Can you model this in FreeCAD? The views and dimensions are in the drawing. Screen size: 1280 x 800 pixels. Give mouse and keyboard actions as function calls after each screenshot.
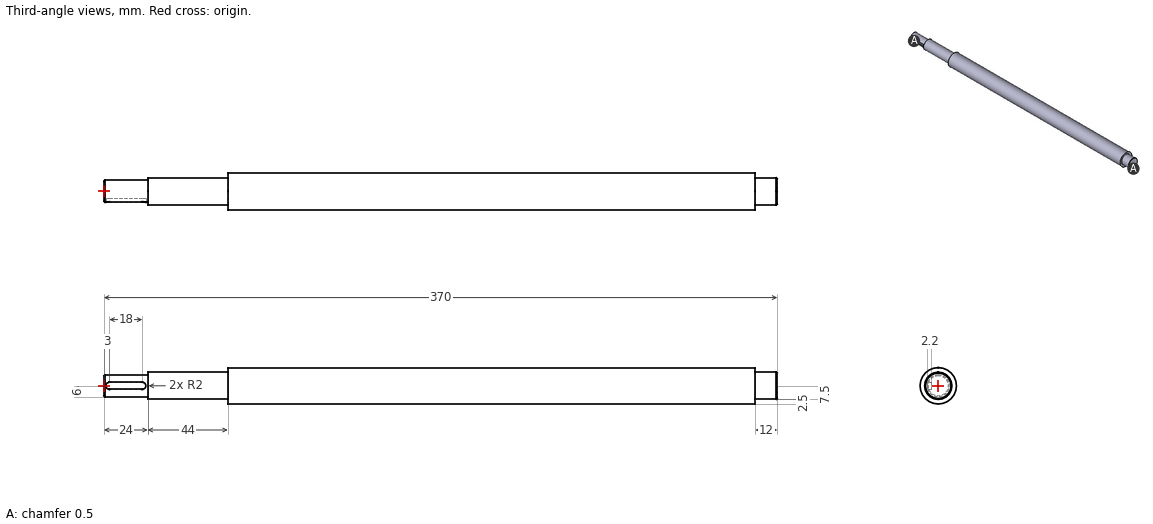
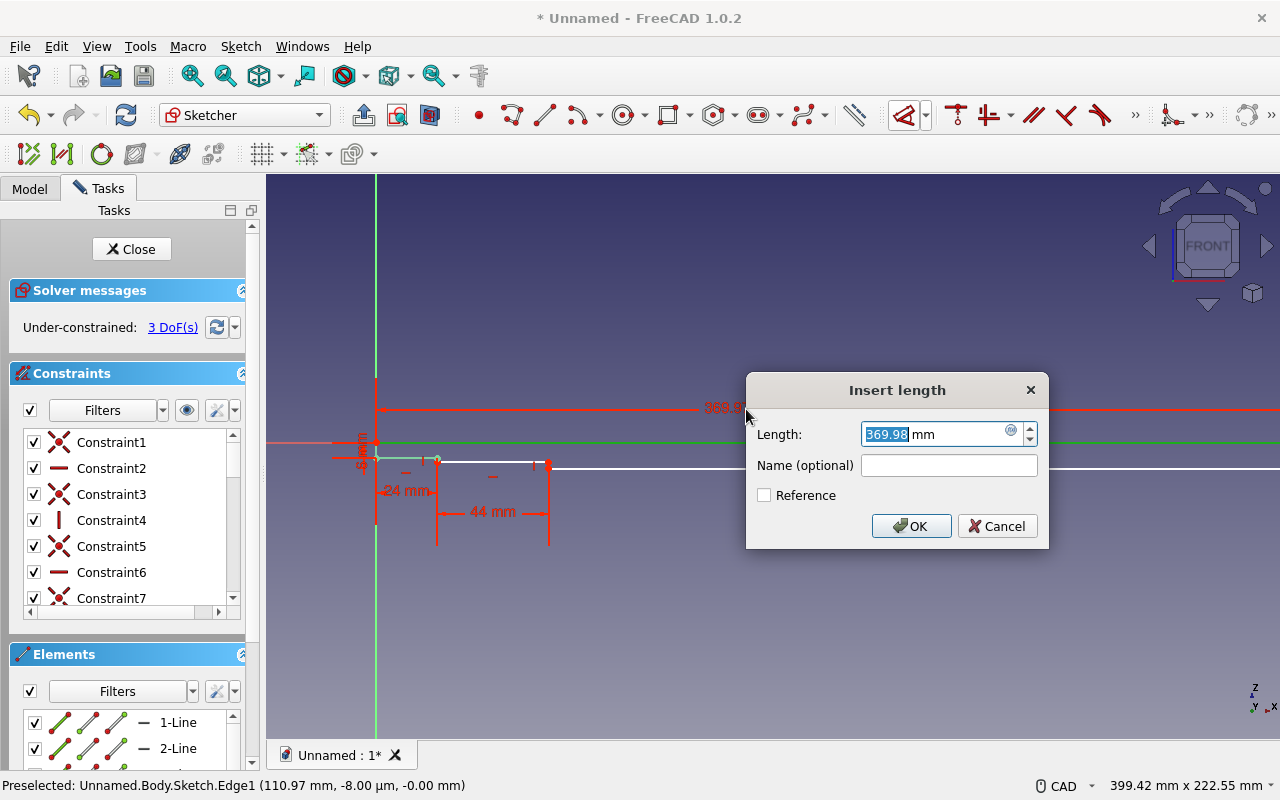
text(370)
key(Return)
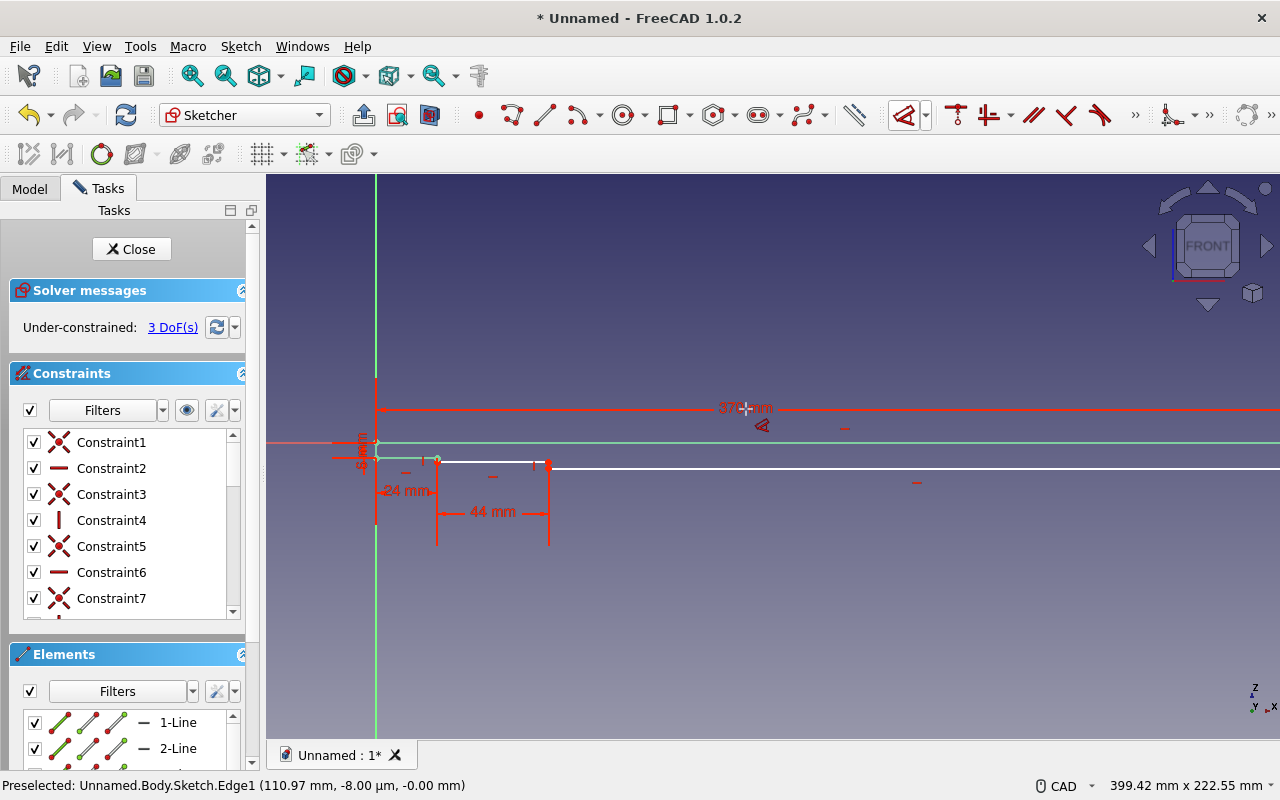
scroll(417, 458, down, 2)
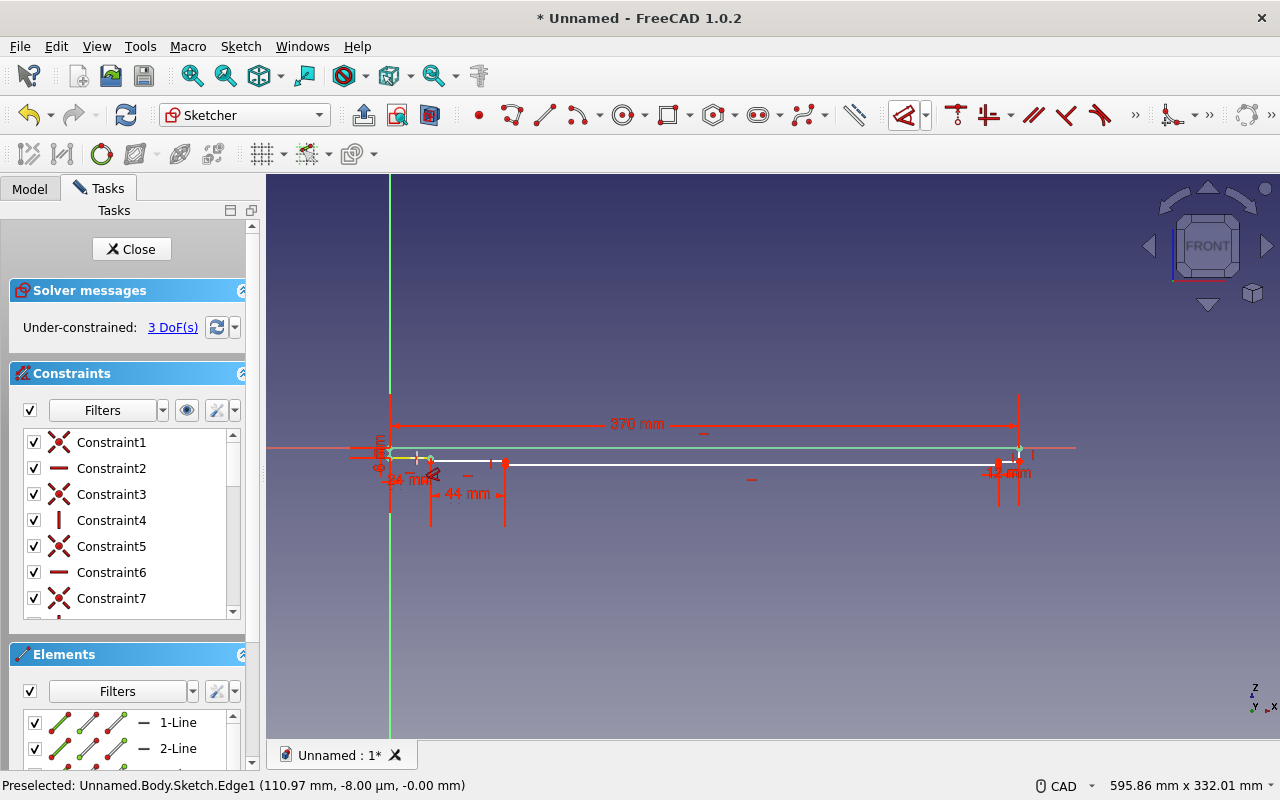
scroll(1019, 455, up, 6)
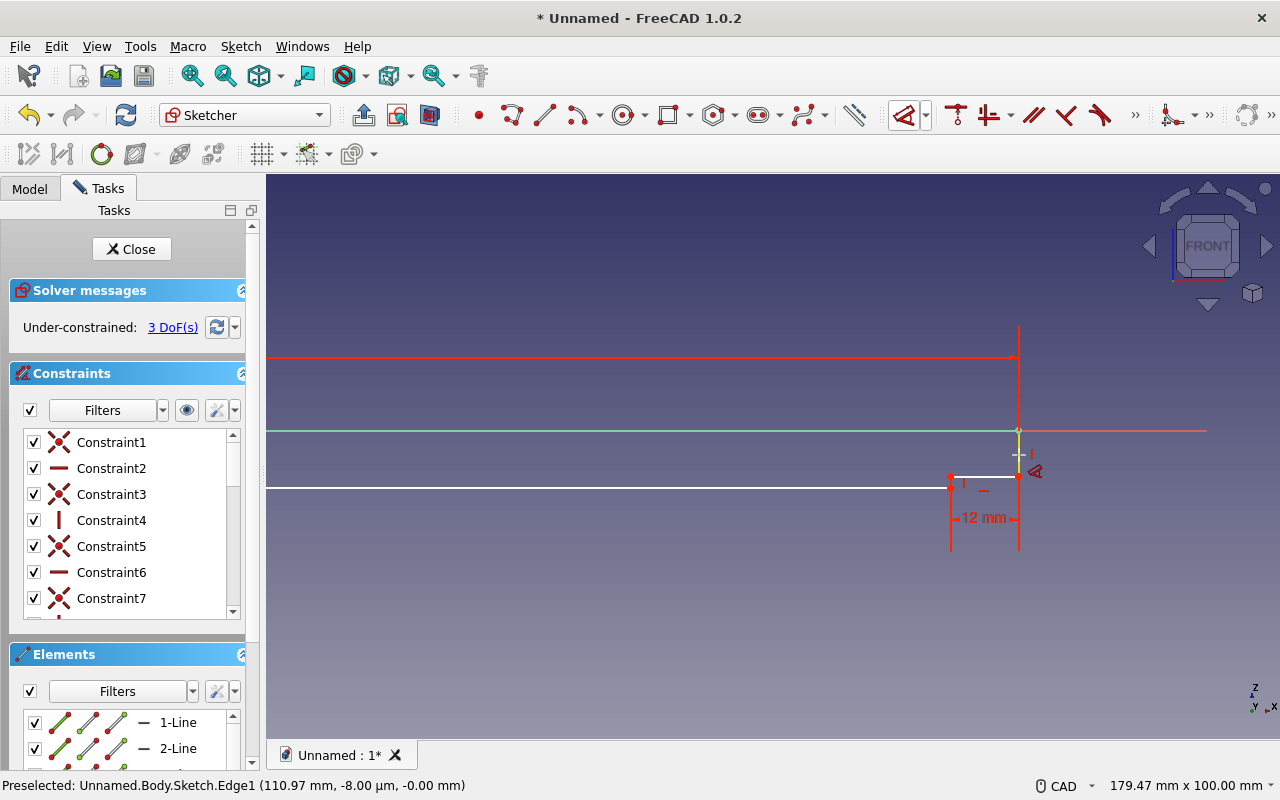
click(1019, 454)
click(1053, 454)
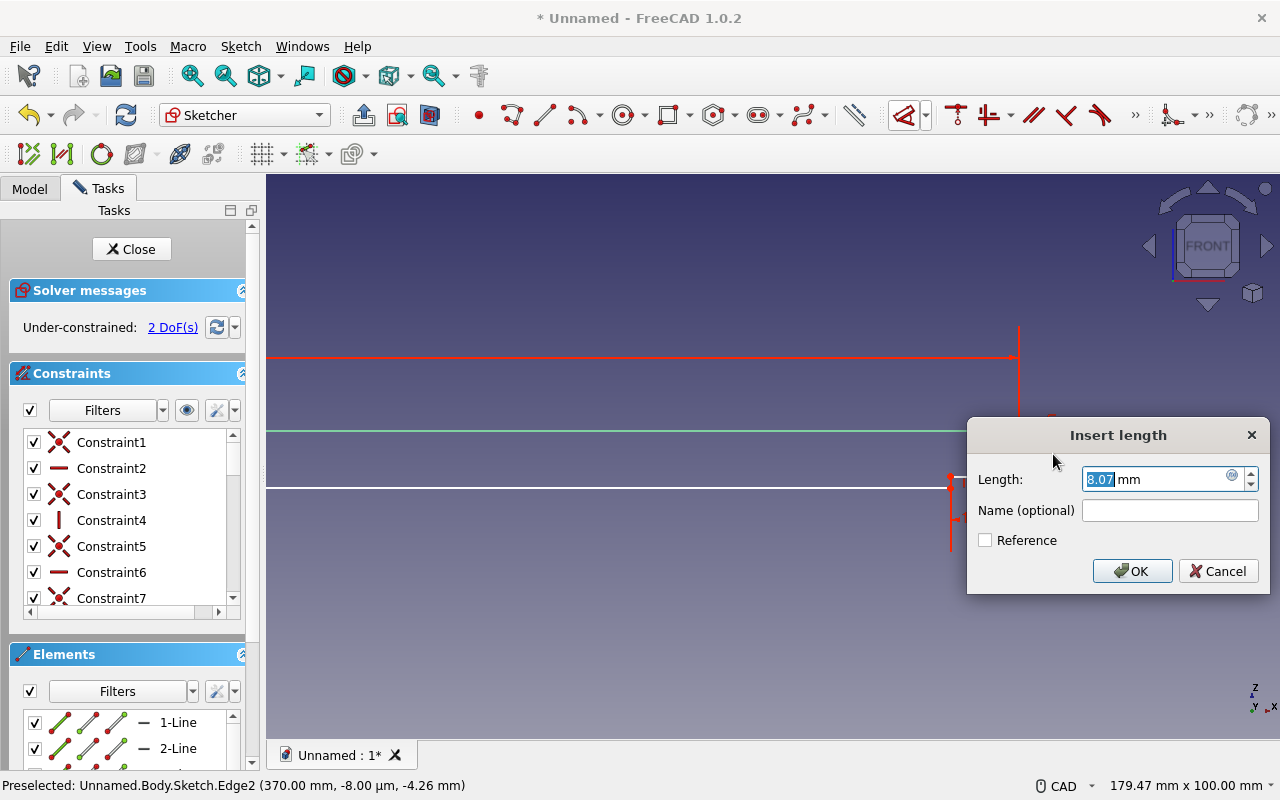
text(7.5)
key(Return)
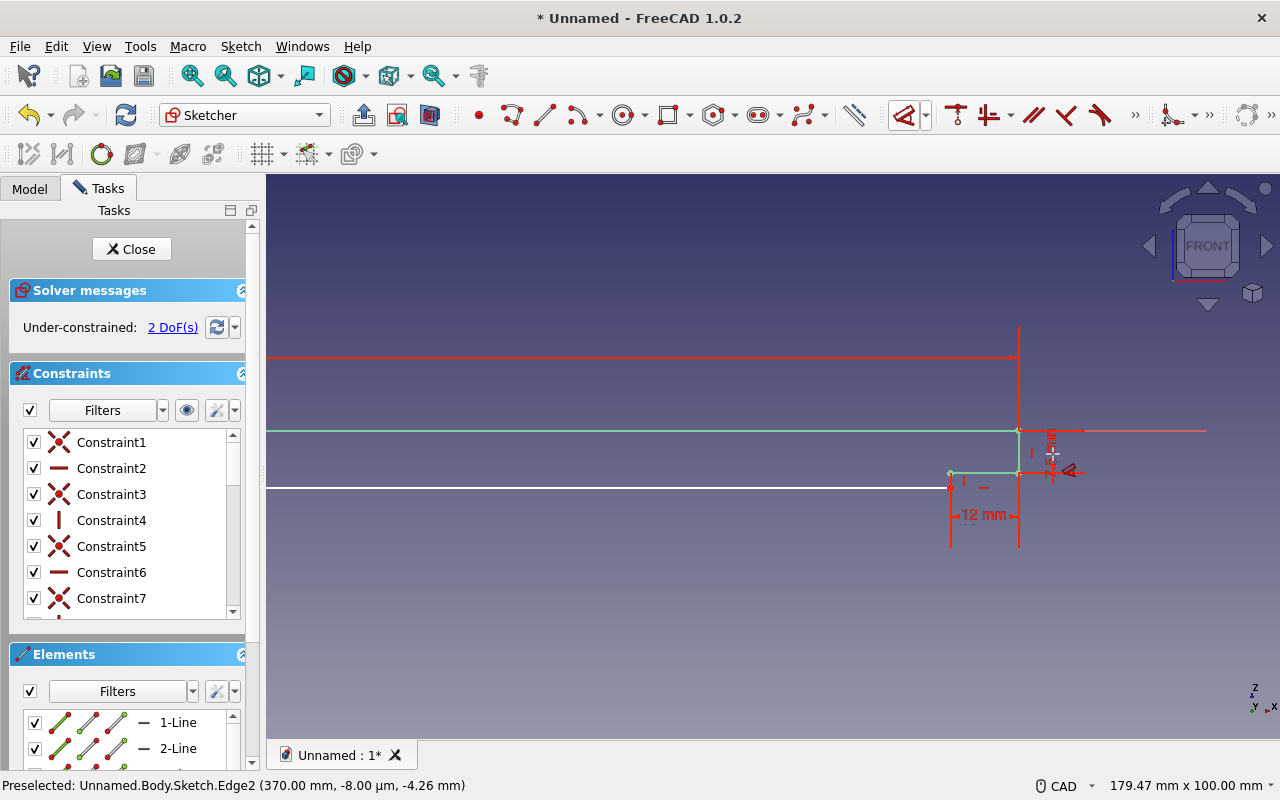
scroll(951, 481, up, 6)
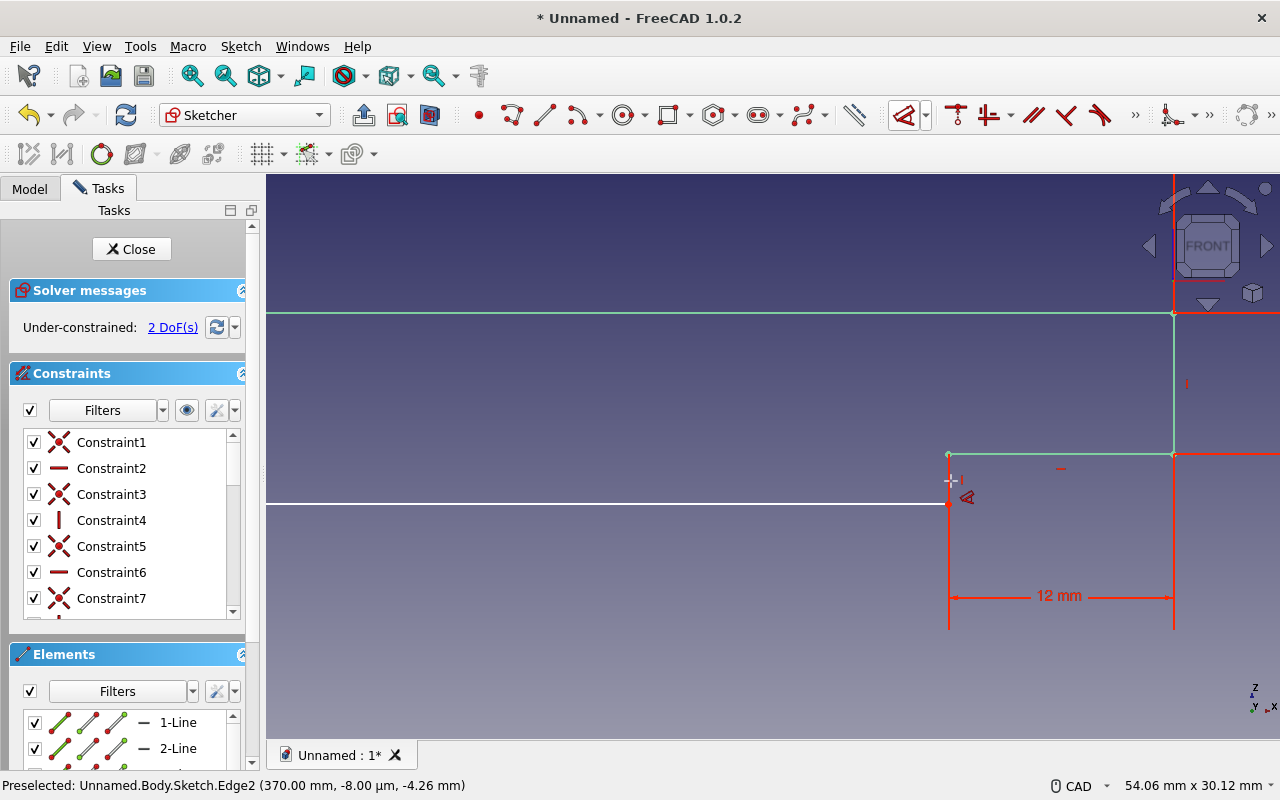
click(949, 479)
click(983, 479)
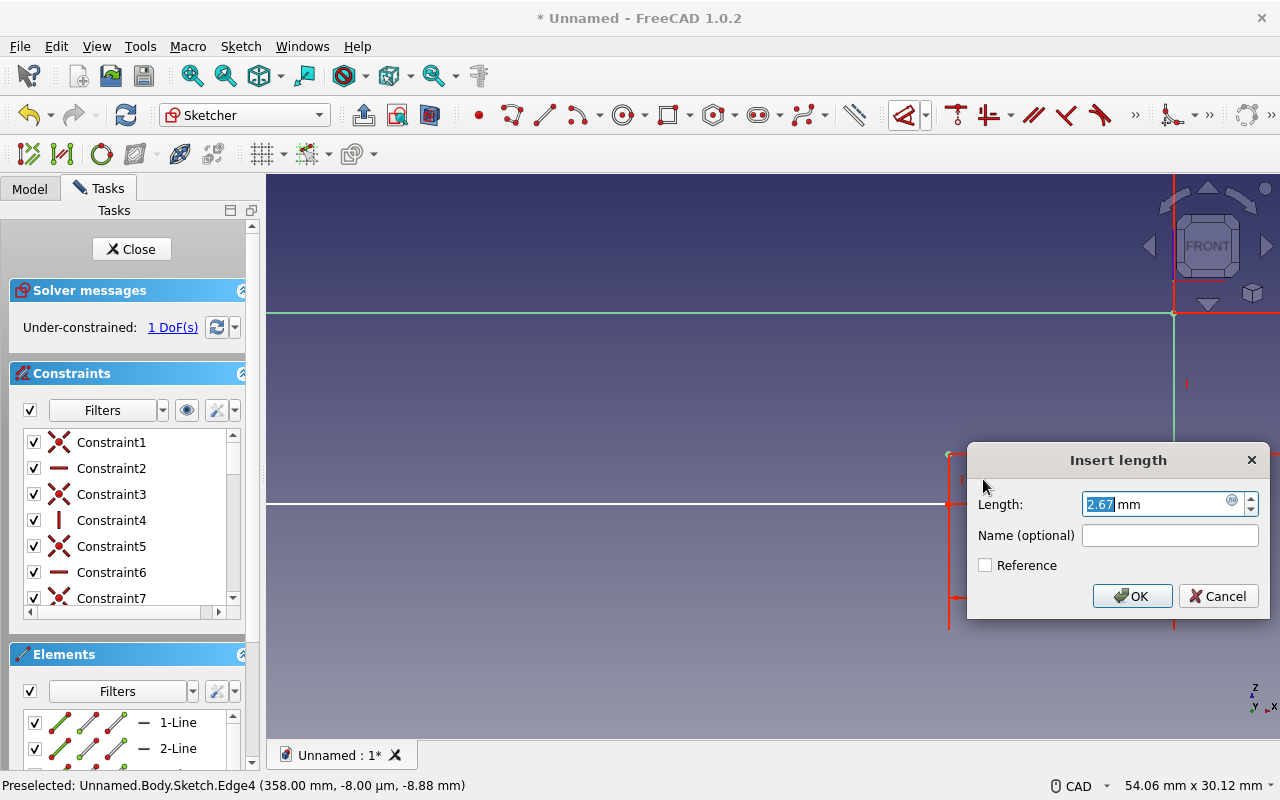
text(2.5)
key(Return)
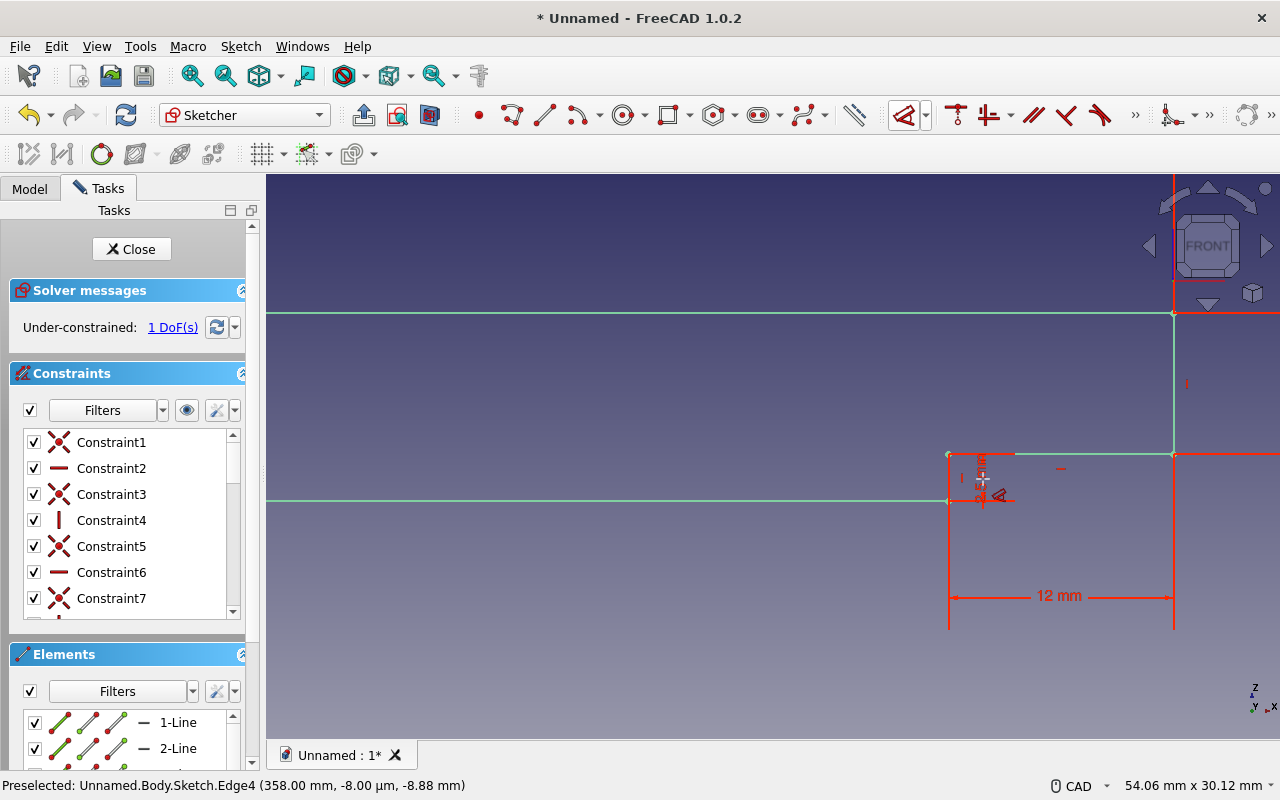
scroll(1004, 461, down, 12)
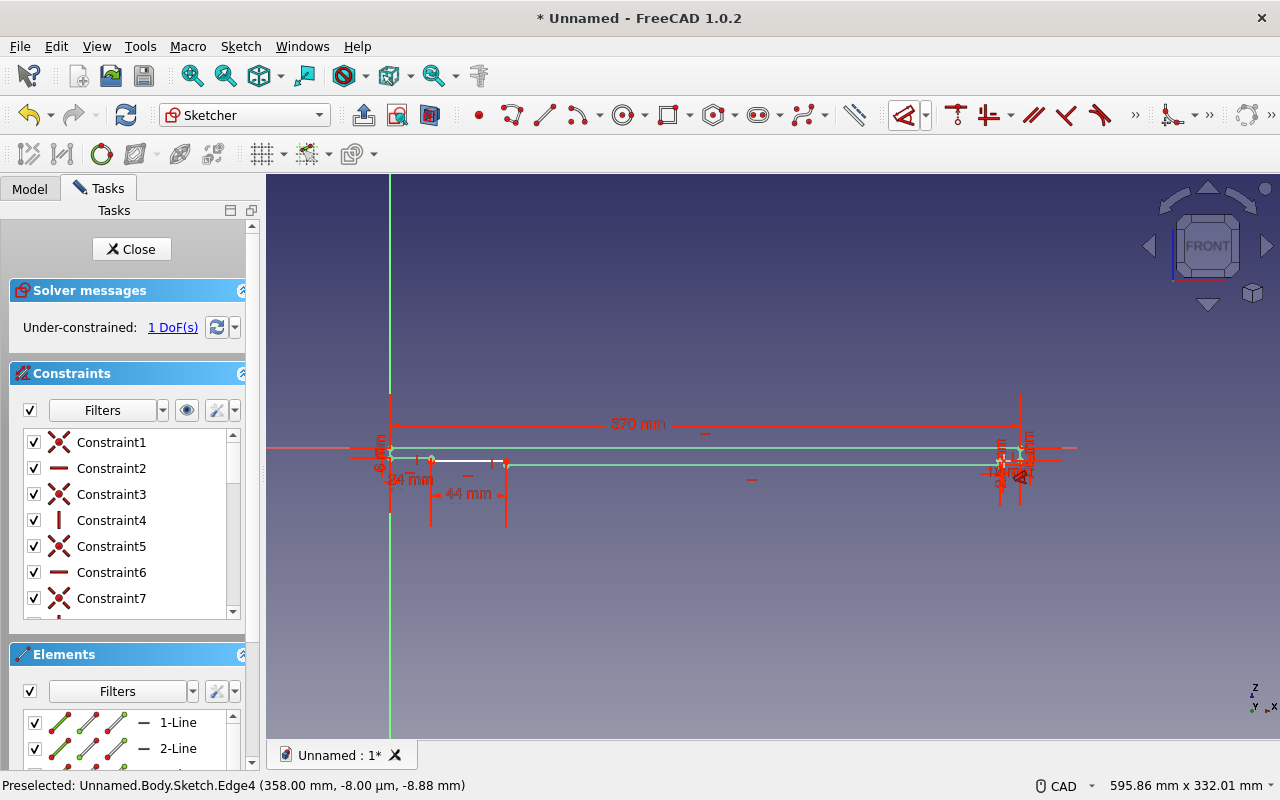
scroll(506, 464, up, 13)